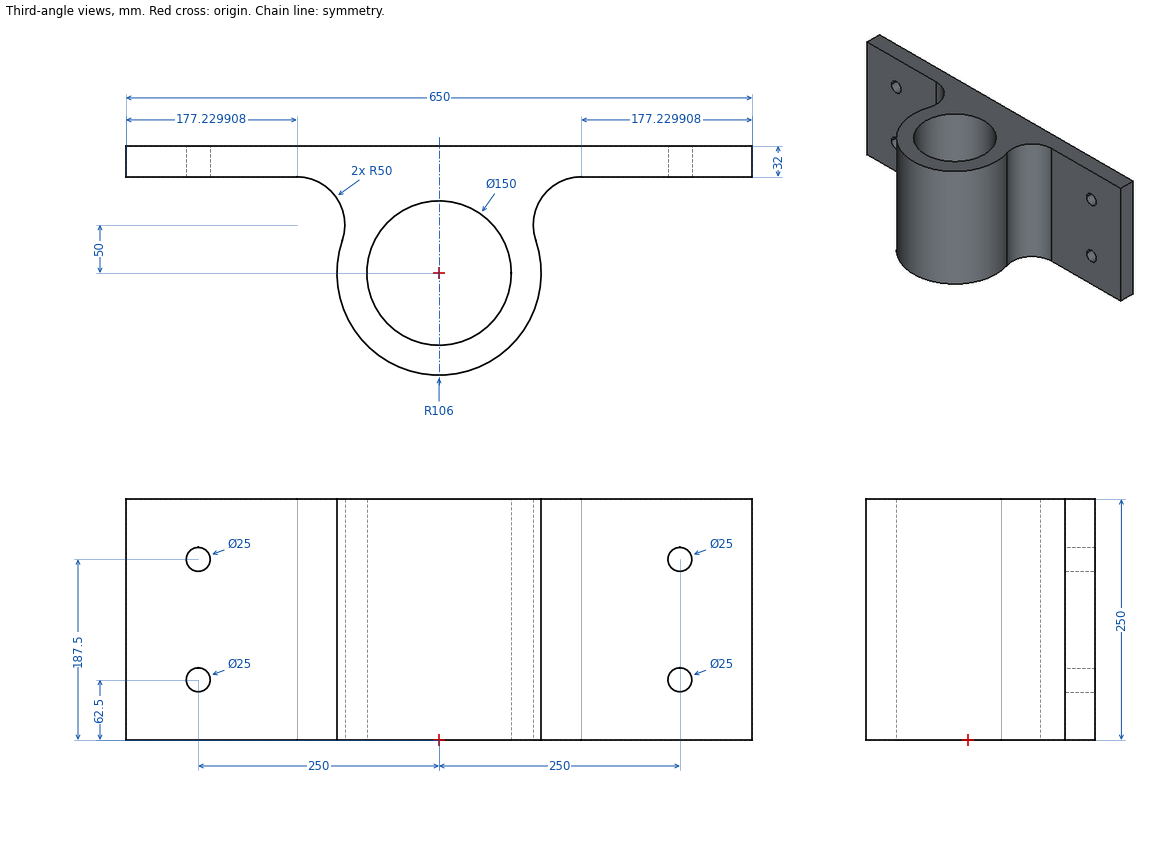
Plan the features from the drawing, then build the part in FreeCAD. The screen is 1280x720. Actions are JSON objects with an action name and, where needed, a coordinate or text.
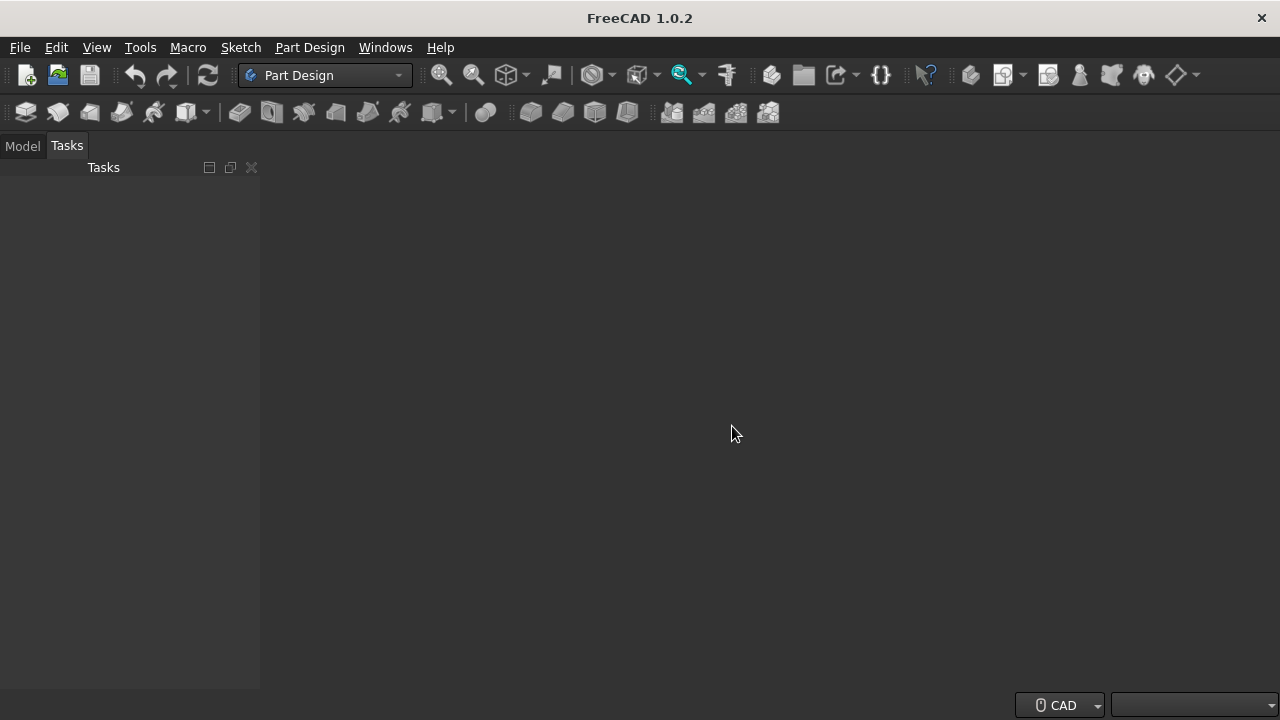
{"action": "left_click", "coordinate": [26, 76]}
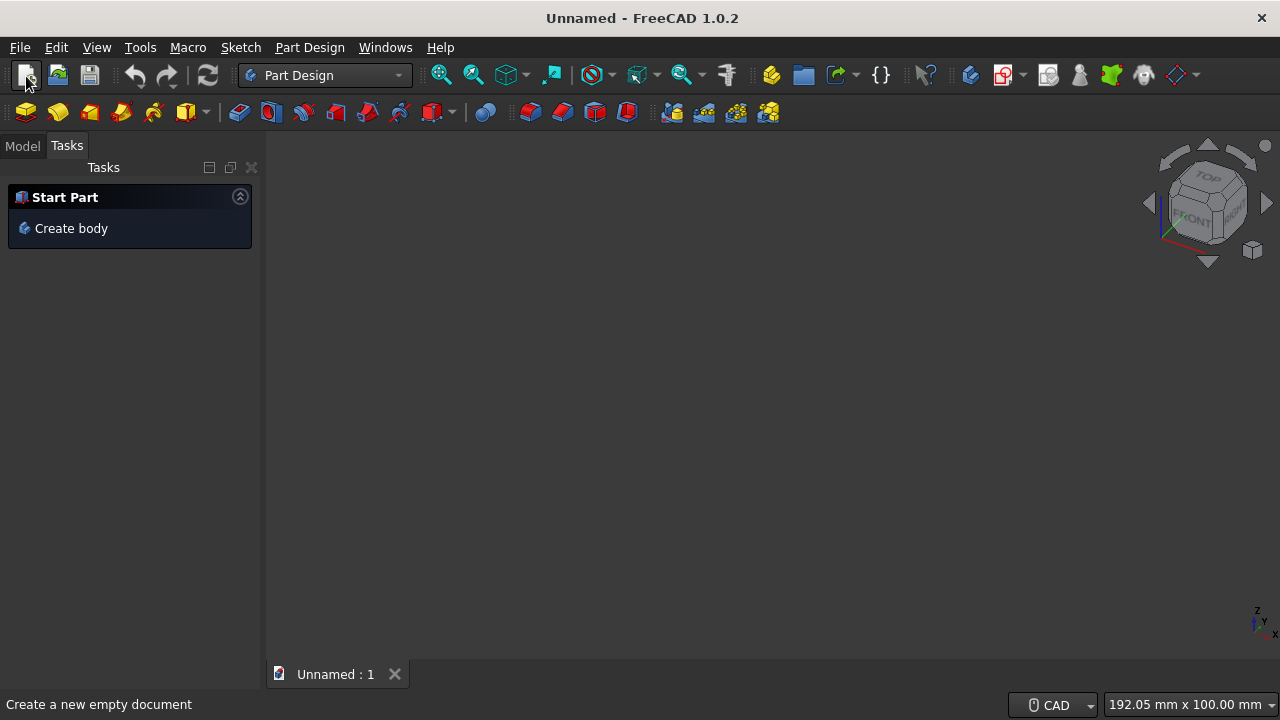
{"action": "left_click", "coordinate": [1004, 76]}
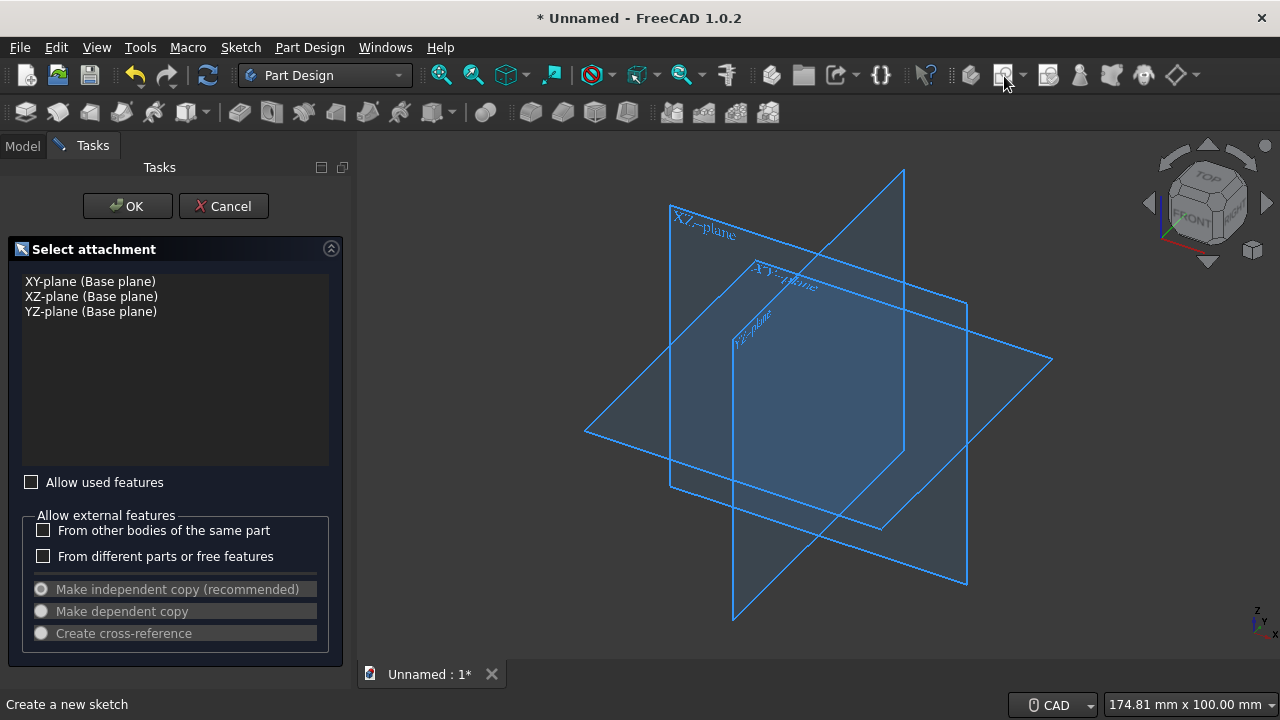
{"action": "left_click", "coordinate": [82, 282]}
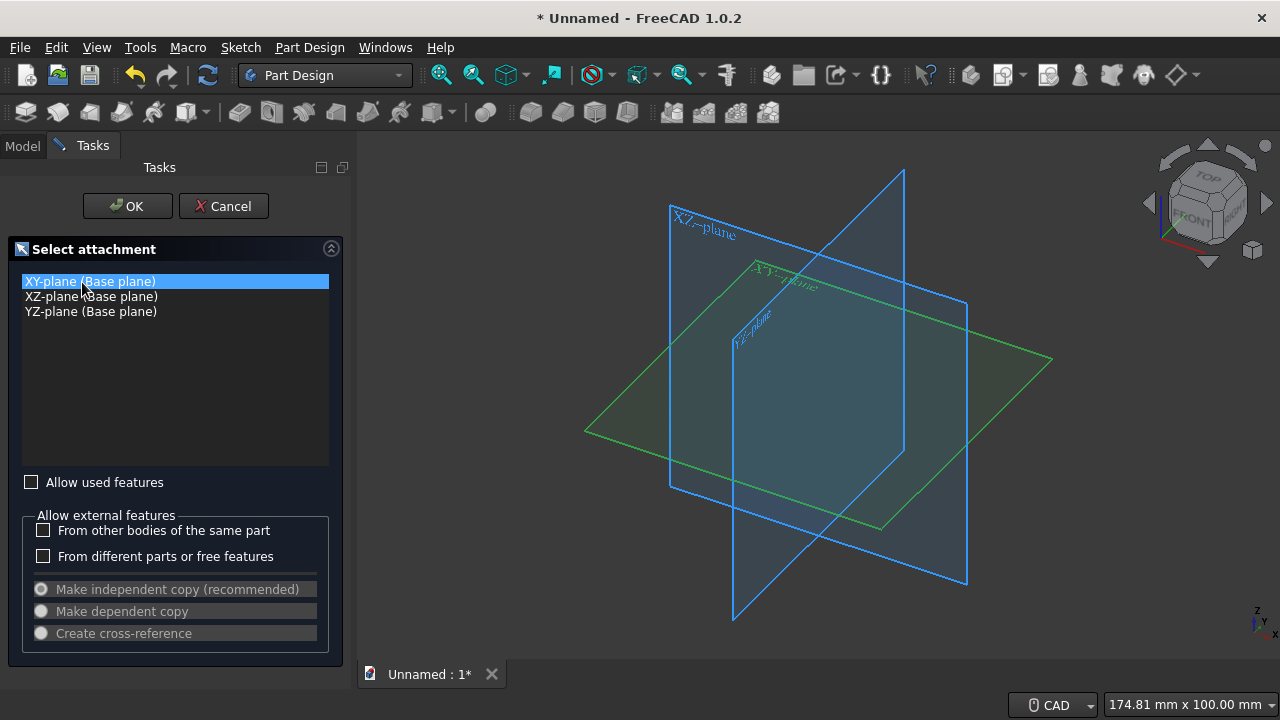
{"action": "left_click", "coordinate": [128, 206]}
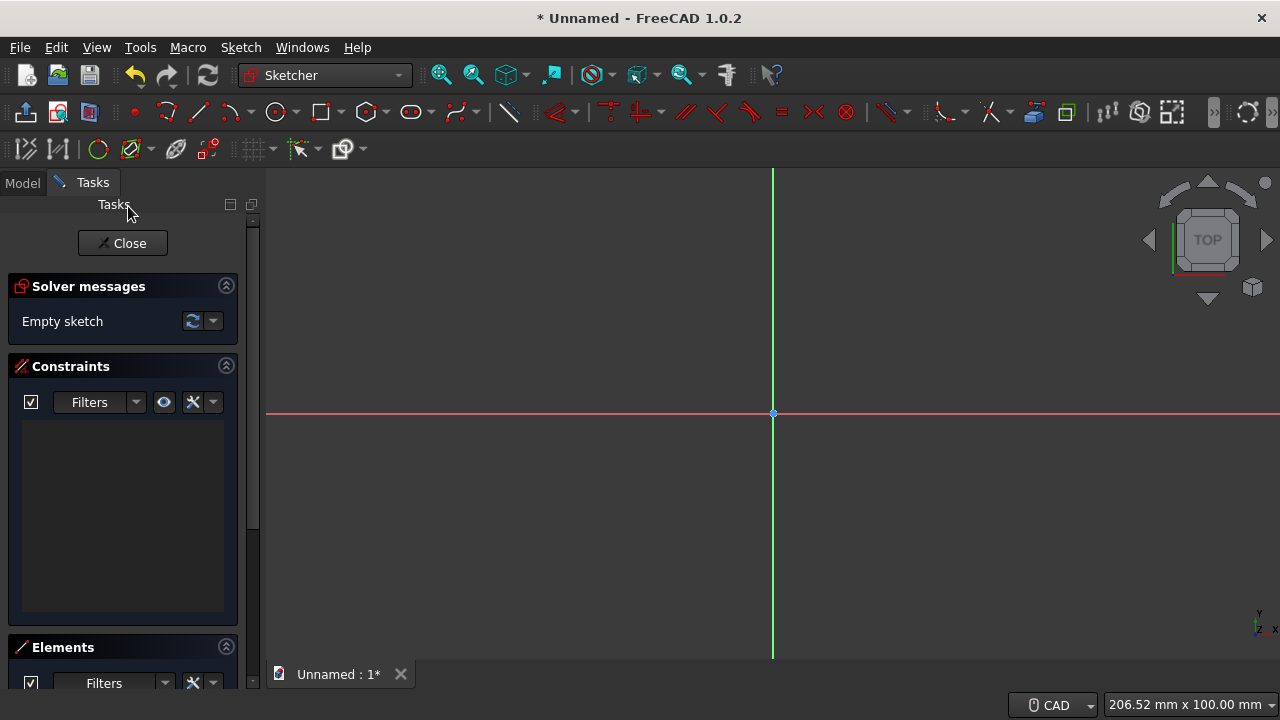
{"action": "scroll", "coordinate": [691, 426], "scroll_direction": "down", "scroll_amount": 9}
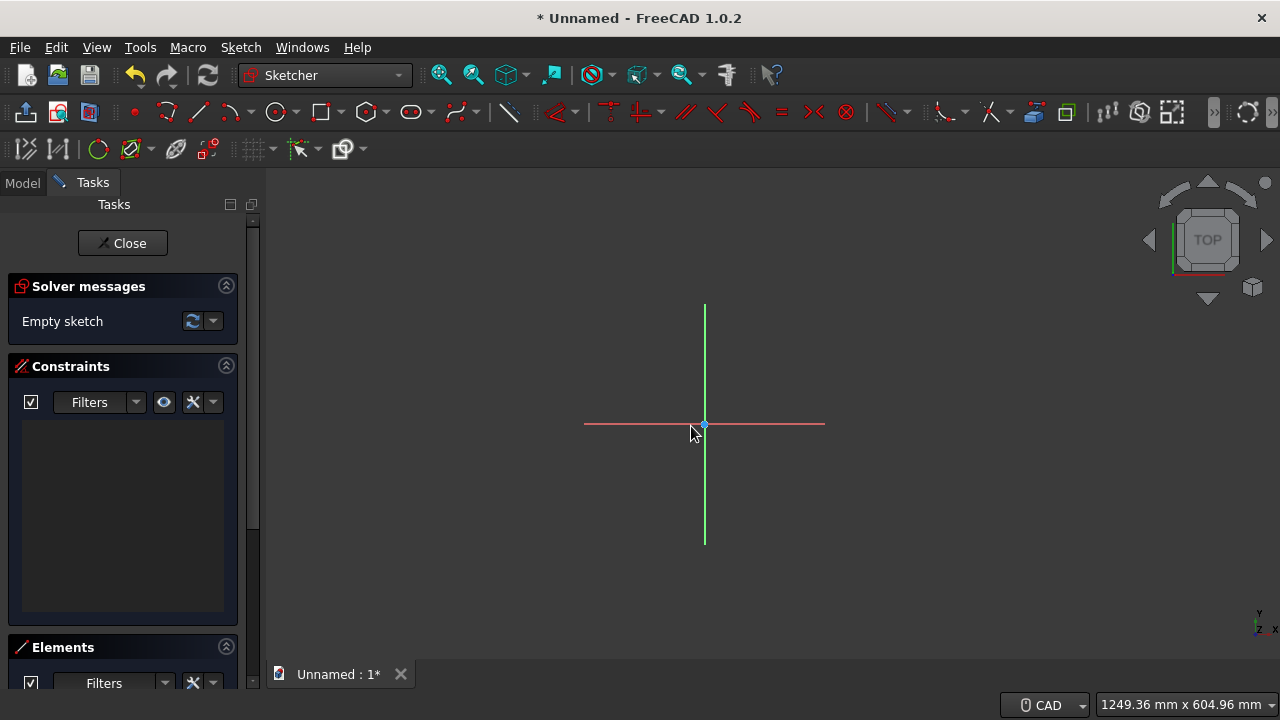
{"action": "left_click", "coordinate": [168, 112]}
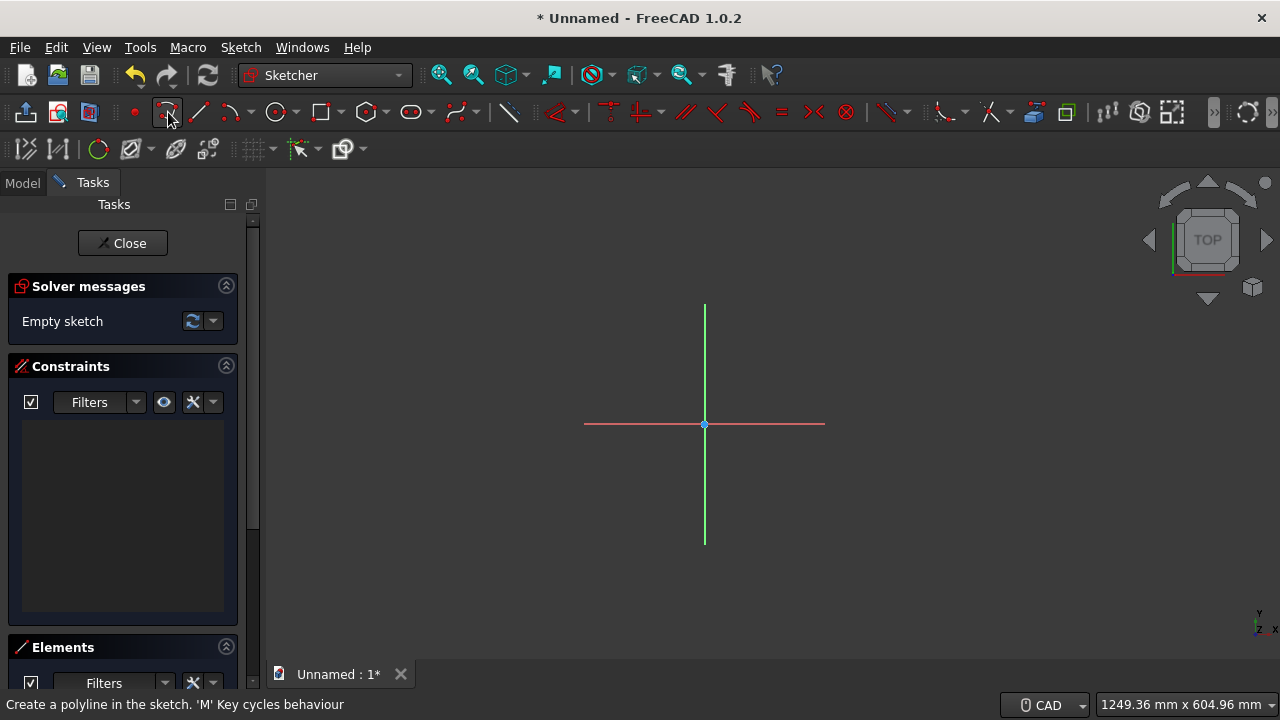
{"action": "left_click", "coordinate": [825, 343]}
{"action": "left_click", "coordinate": [969, 343]}
{"action": "left_click", "coordinate": [969, 317]}
{"action": "left_click", "coordinate": [441, 317]}
{"action": "left_click", "coordinate": [441, 343]}
{"action": "left_click", "coordinate": [585, 343]}
{"action": "right_click", "coordinate": [585, 343]}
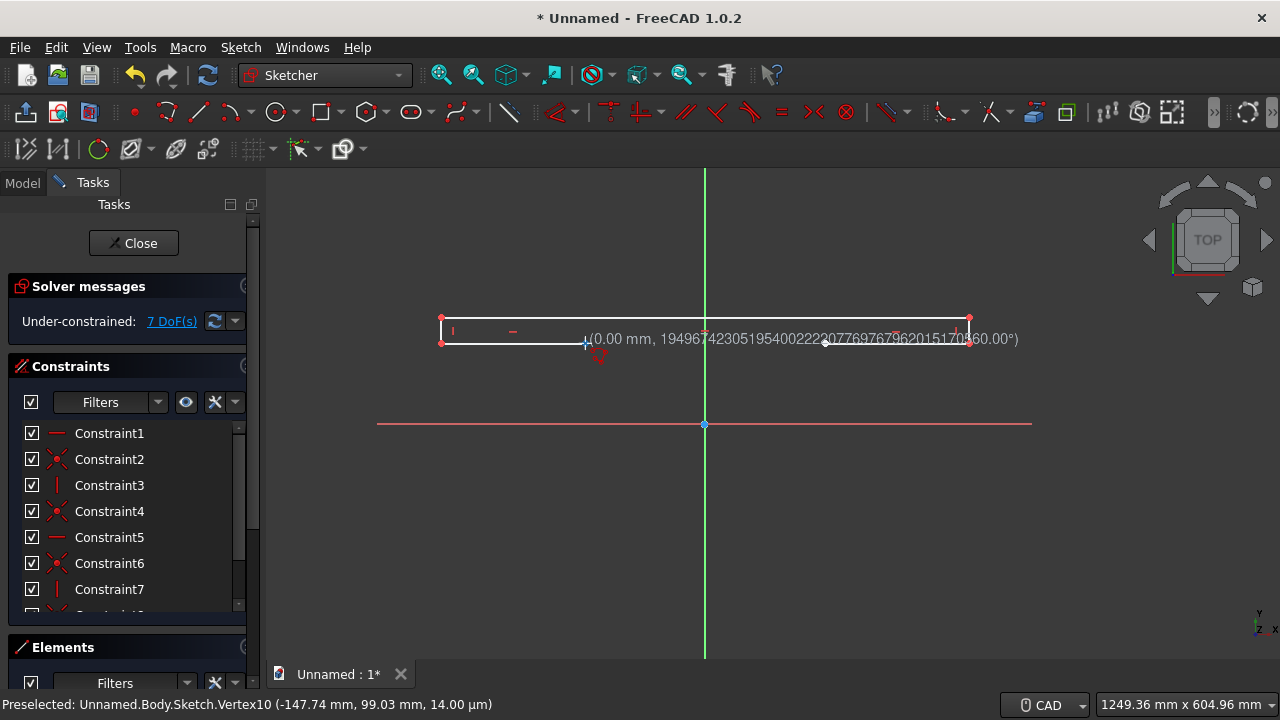
{"action": "left_click", "coordinate": [254, 112]}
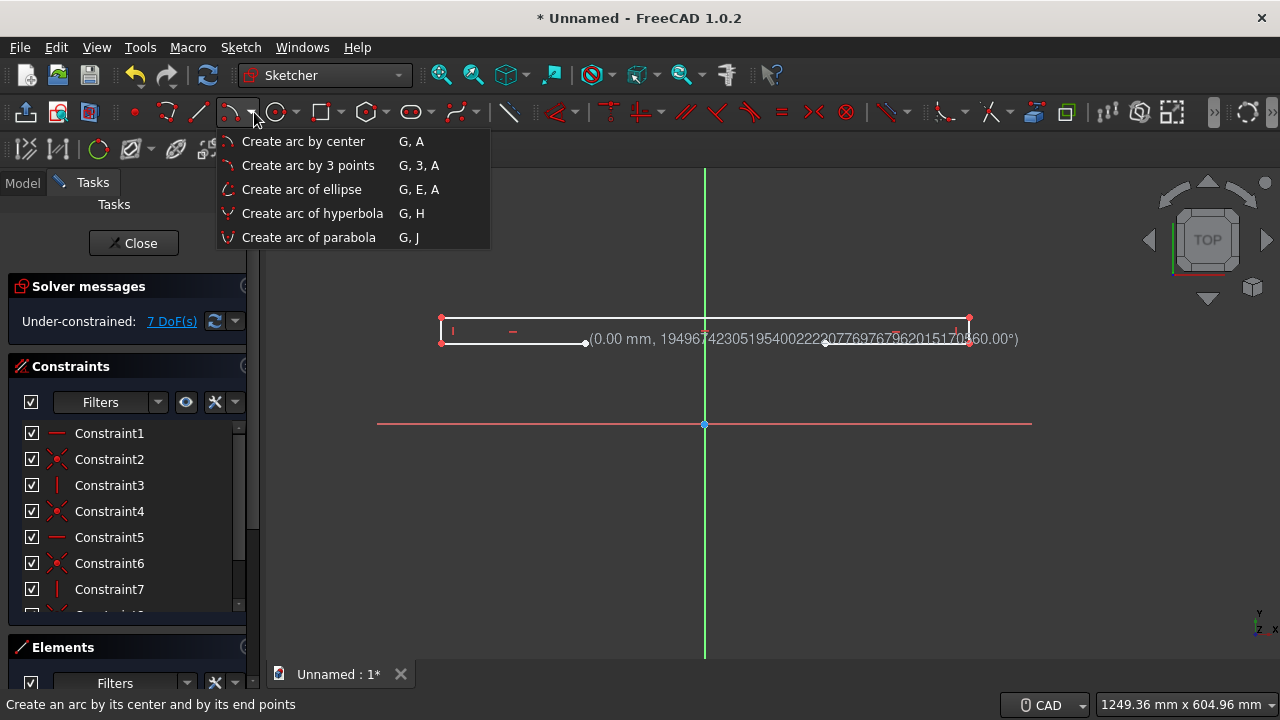
{"action": "left_click", "coordinate": [354, 165]}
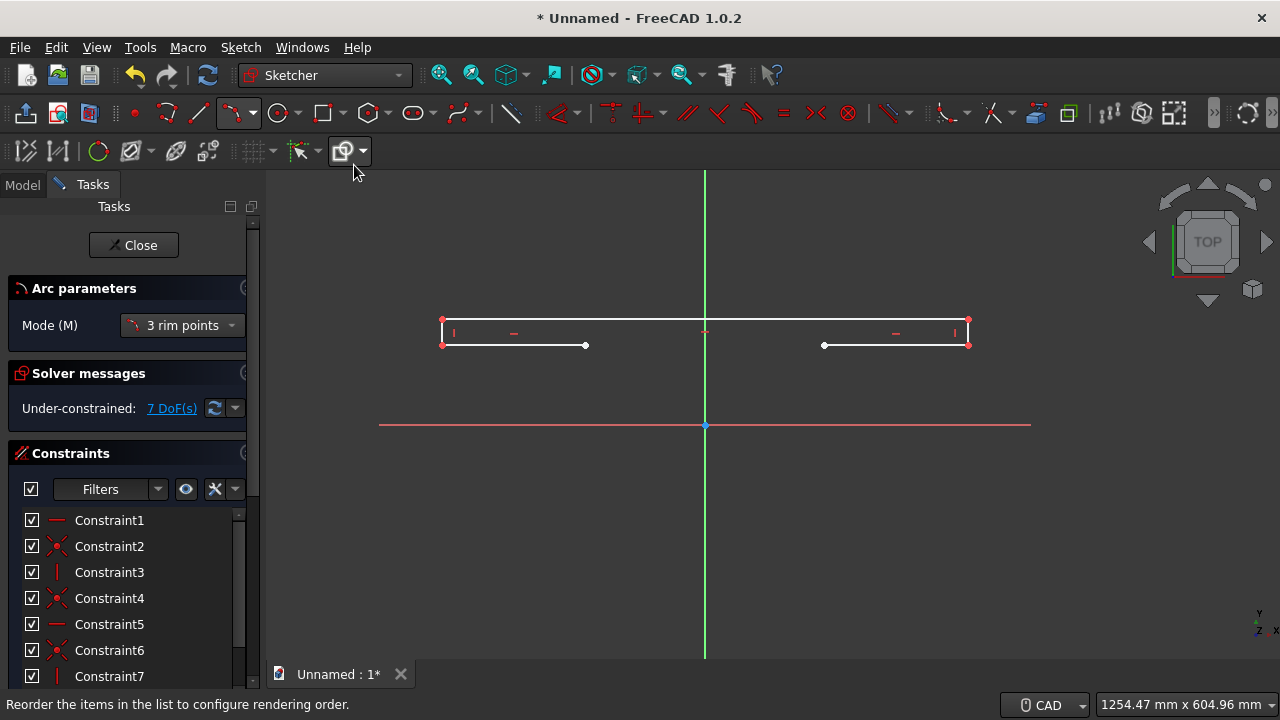
{"action": "left_click", "coordinate": [586, 345]}
{"action": "left_click", "coordinate": [624, 398]}
{"action": "left_click", "coordinate": [619, 361]}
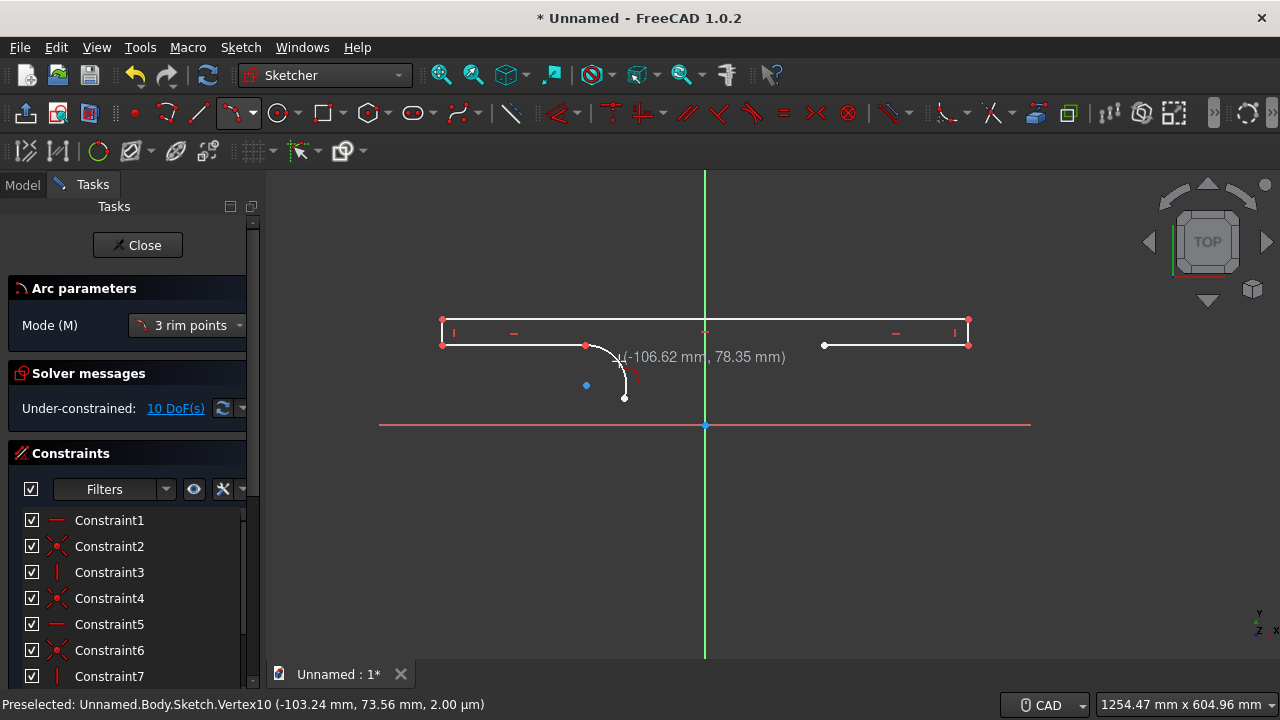
{"action": "left_click", "coordinate": [624, 399]}
{"action": "left_click", "coordinate": [786, 398]}
{"action": "left_click", "coordinate": [673, 505]}